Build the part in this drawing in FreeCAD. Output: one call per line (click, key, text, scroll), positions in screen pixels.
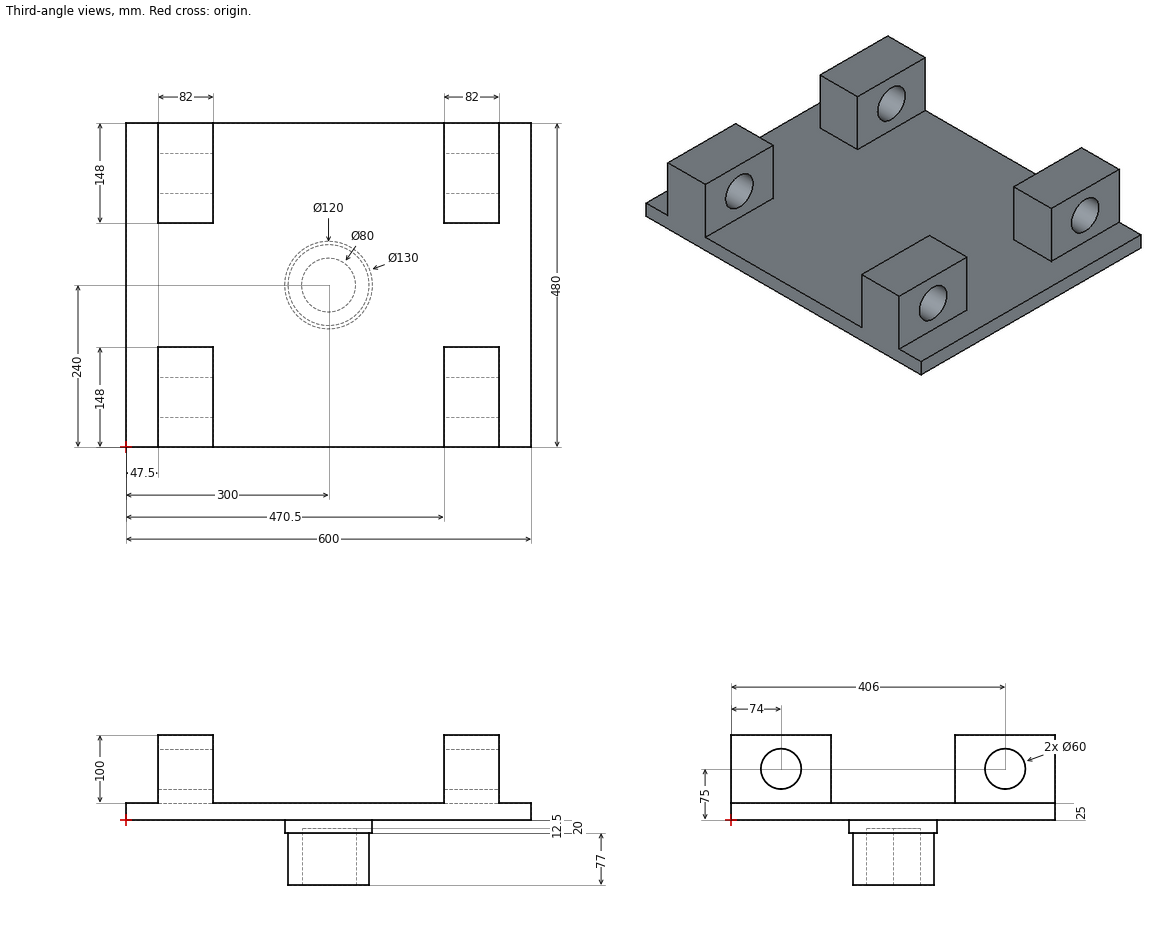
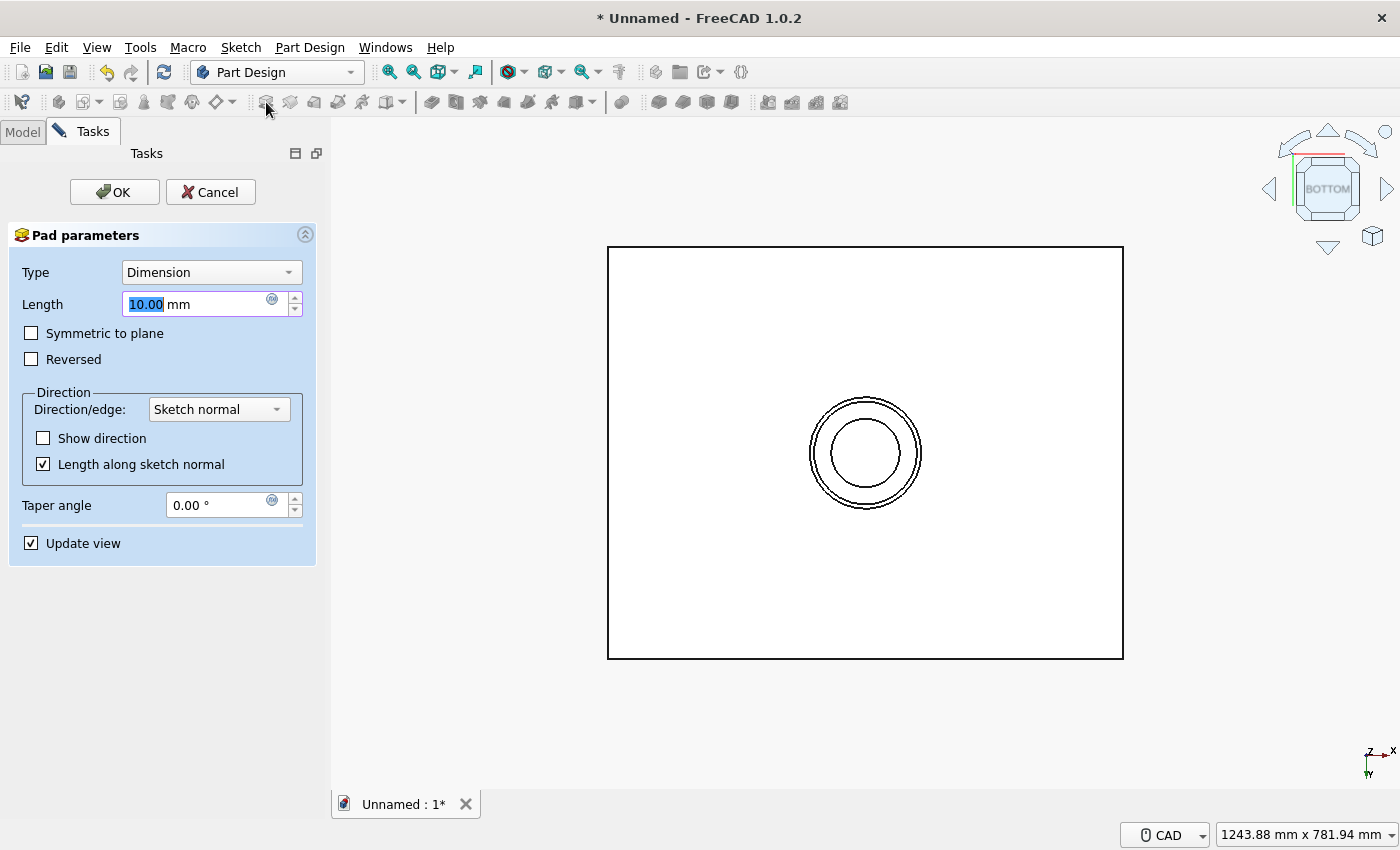
text(12.5)
key(Tab)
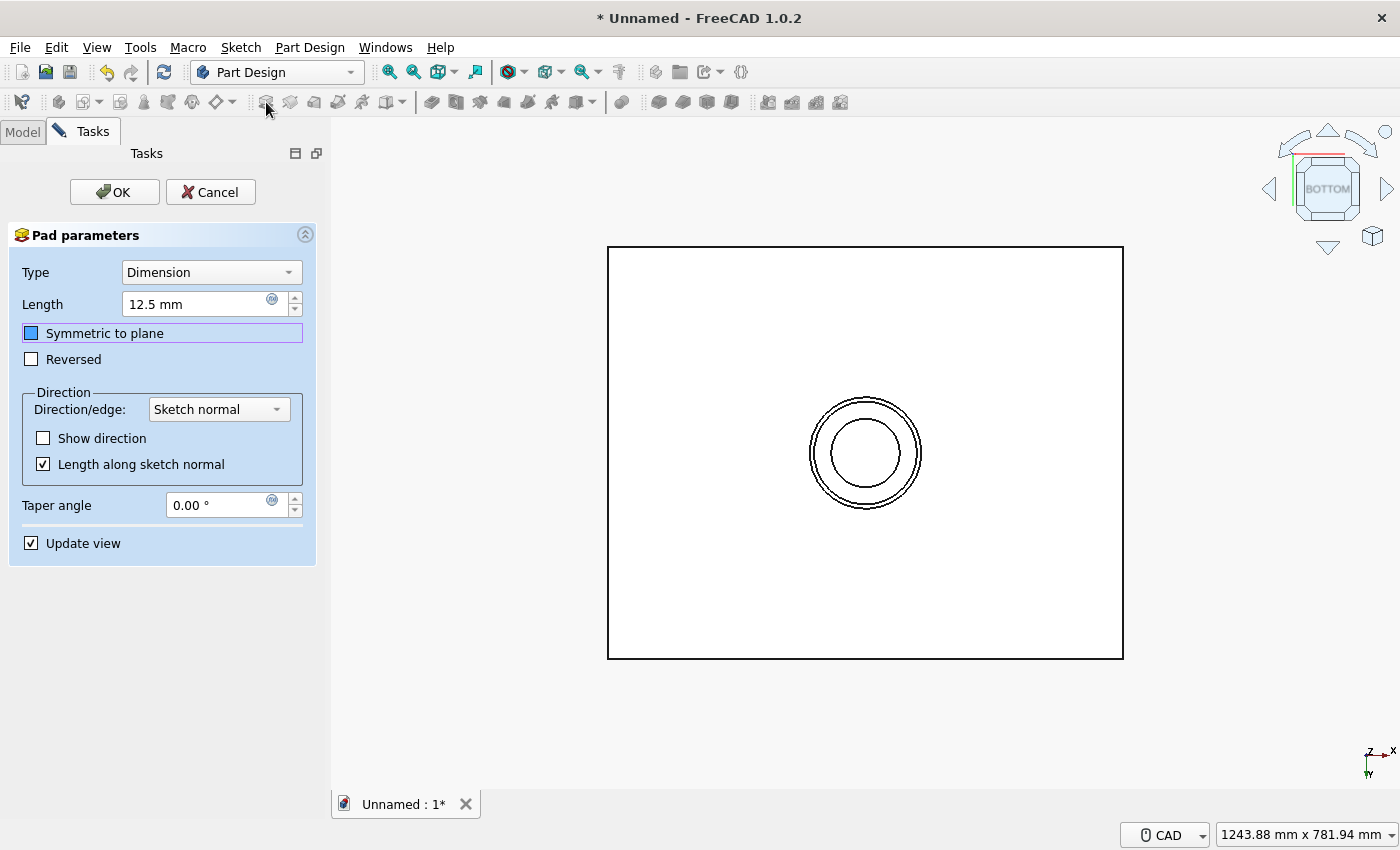
click(115, 192)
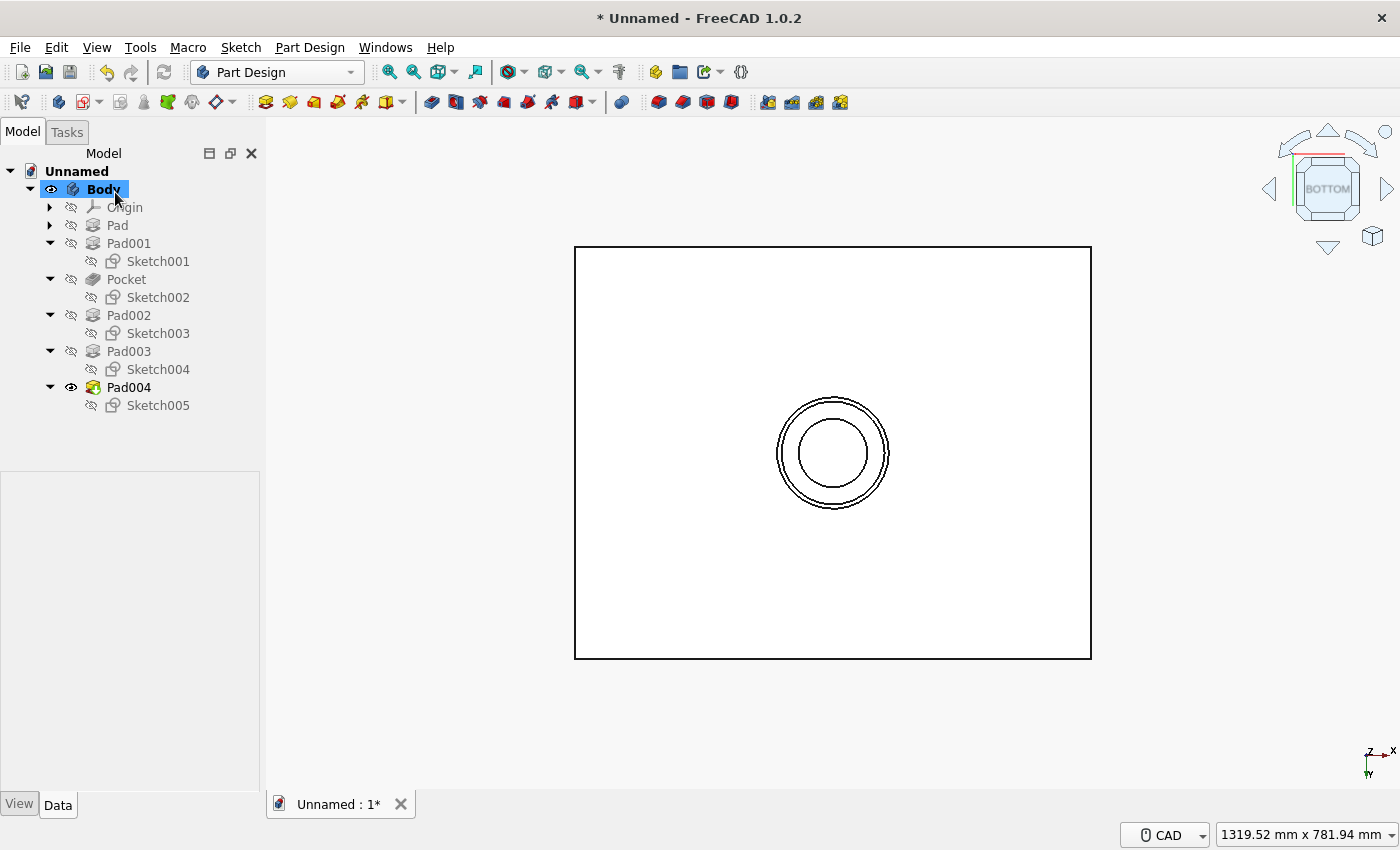
key(0)